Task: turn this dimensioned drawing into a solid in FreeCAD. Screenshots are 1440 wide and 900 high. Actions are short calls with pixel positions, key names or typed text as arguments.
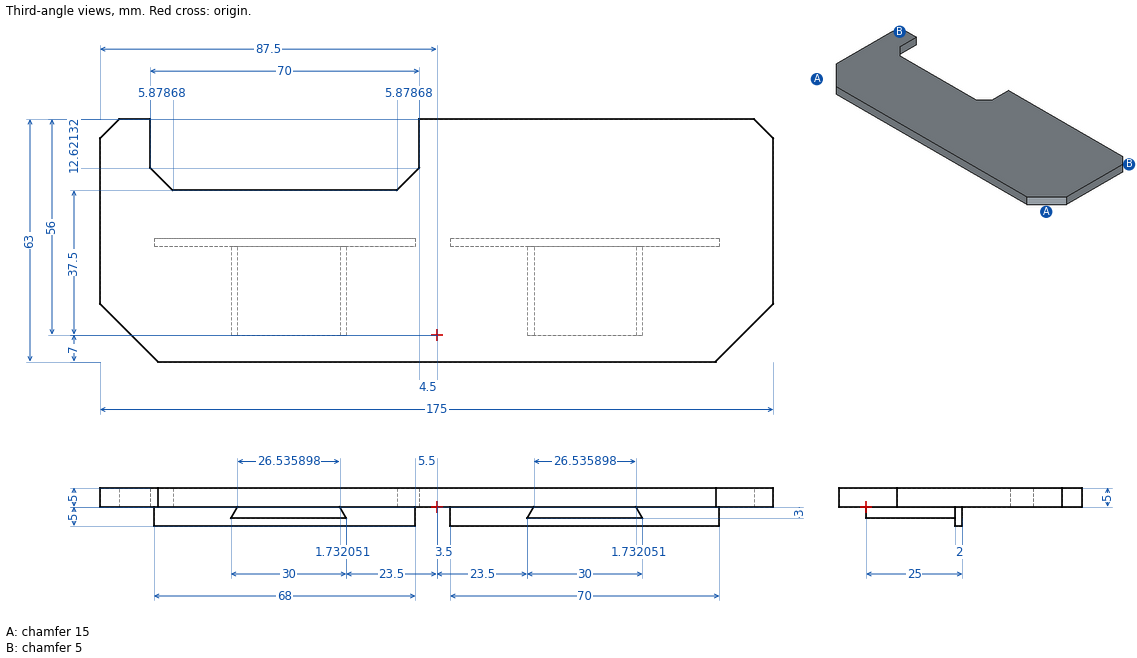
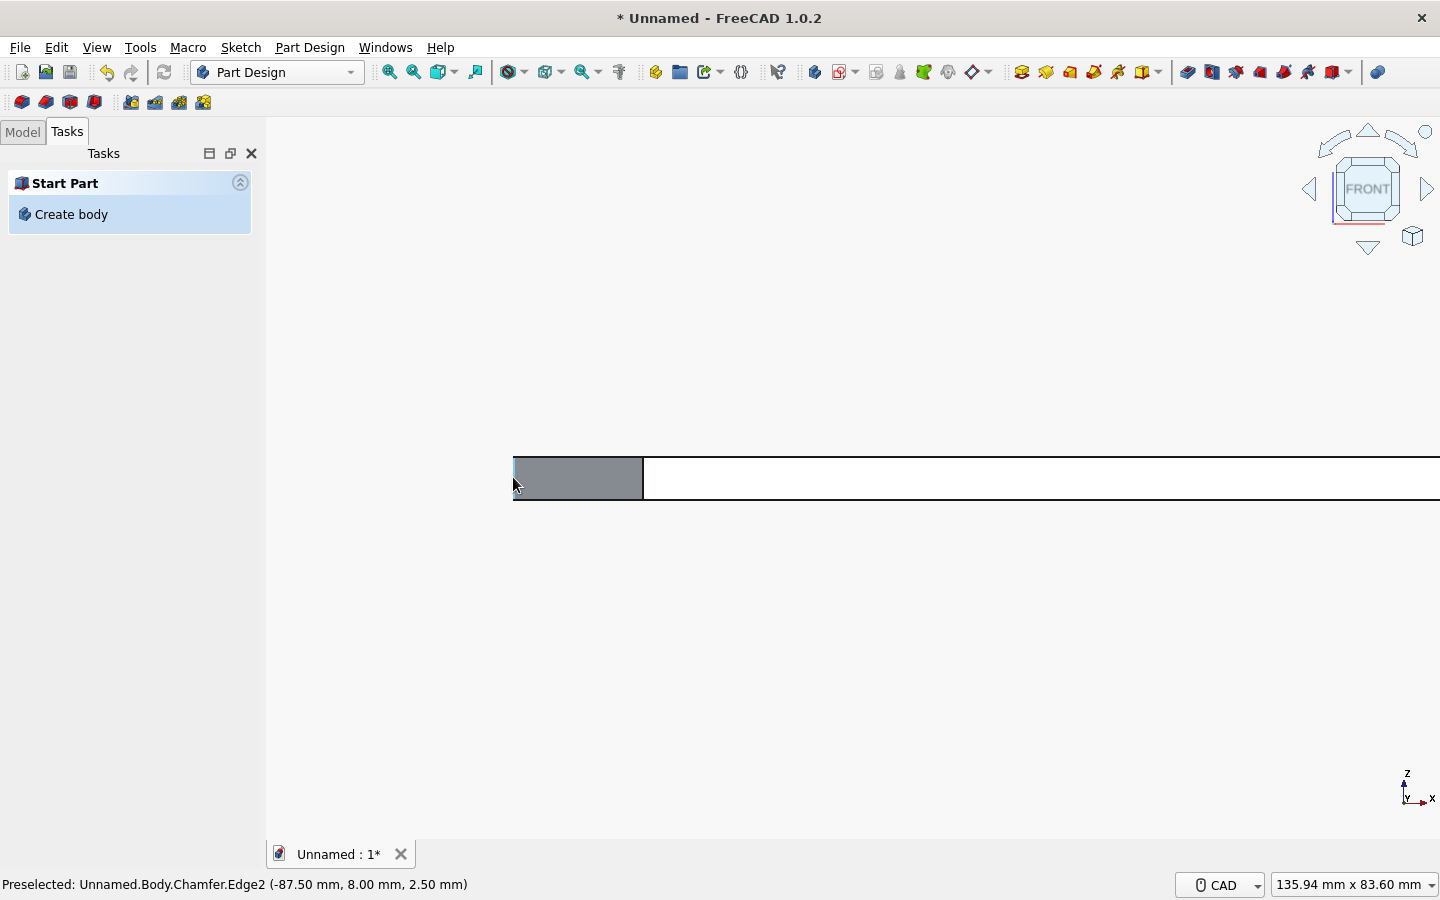
key(v)
key(f)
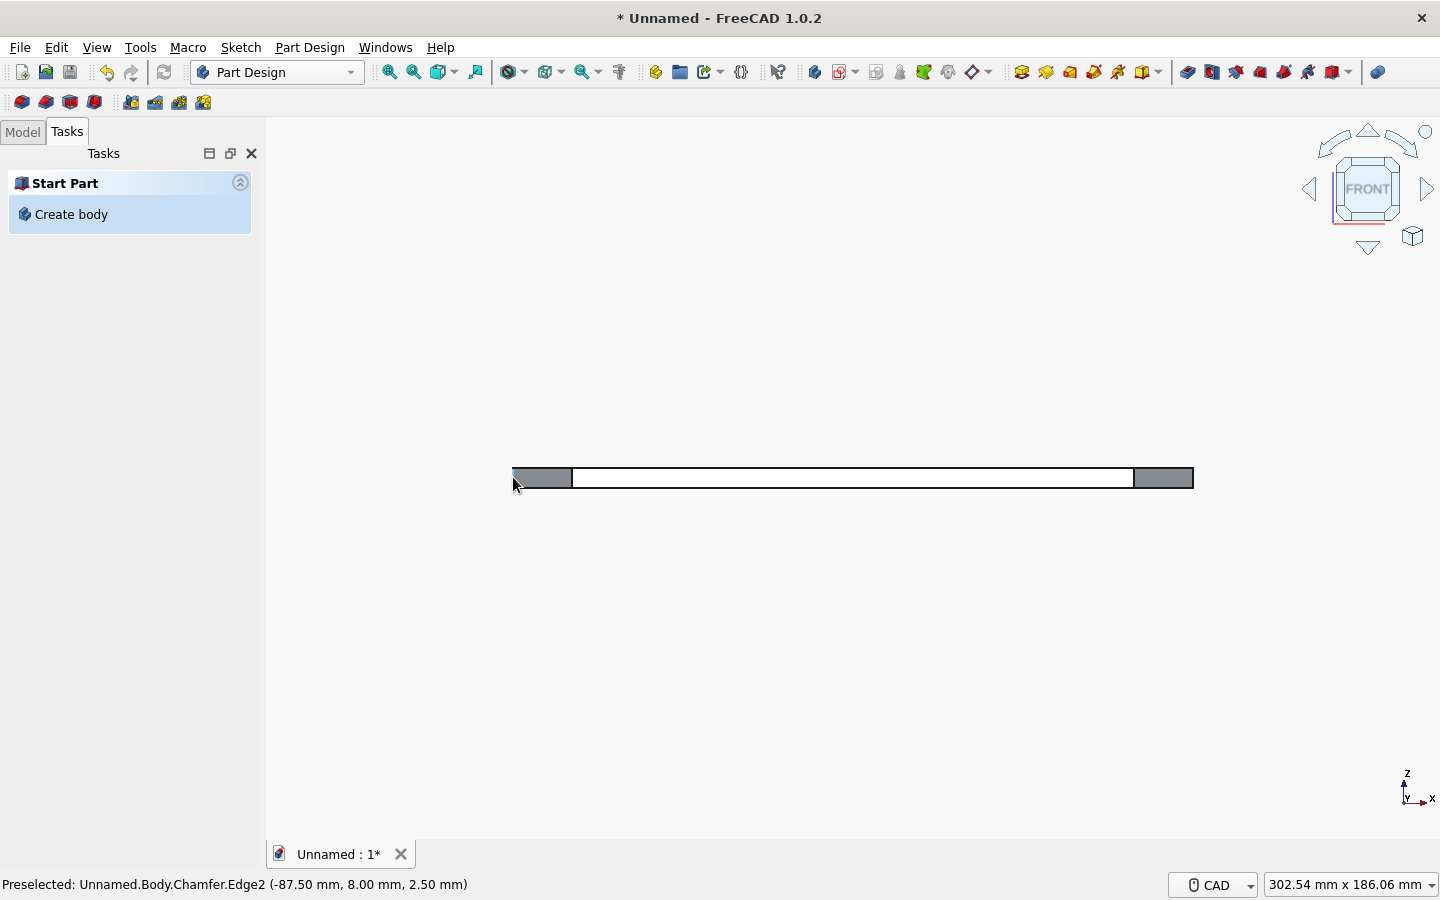
key(0)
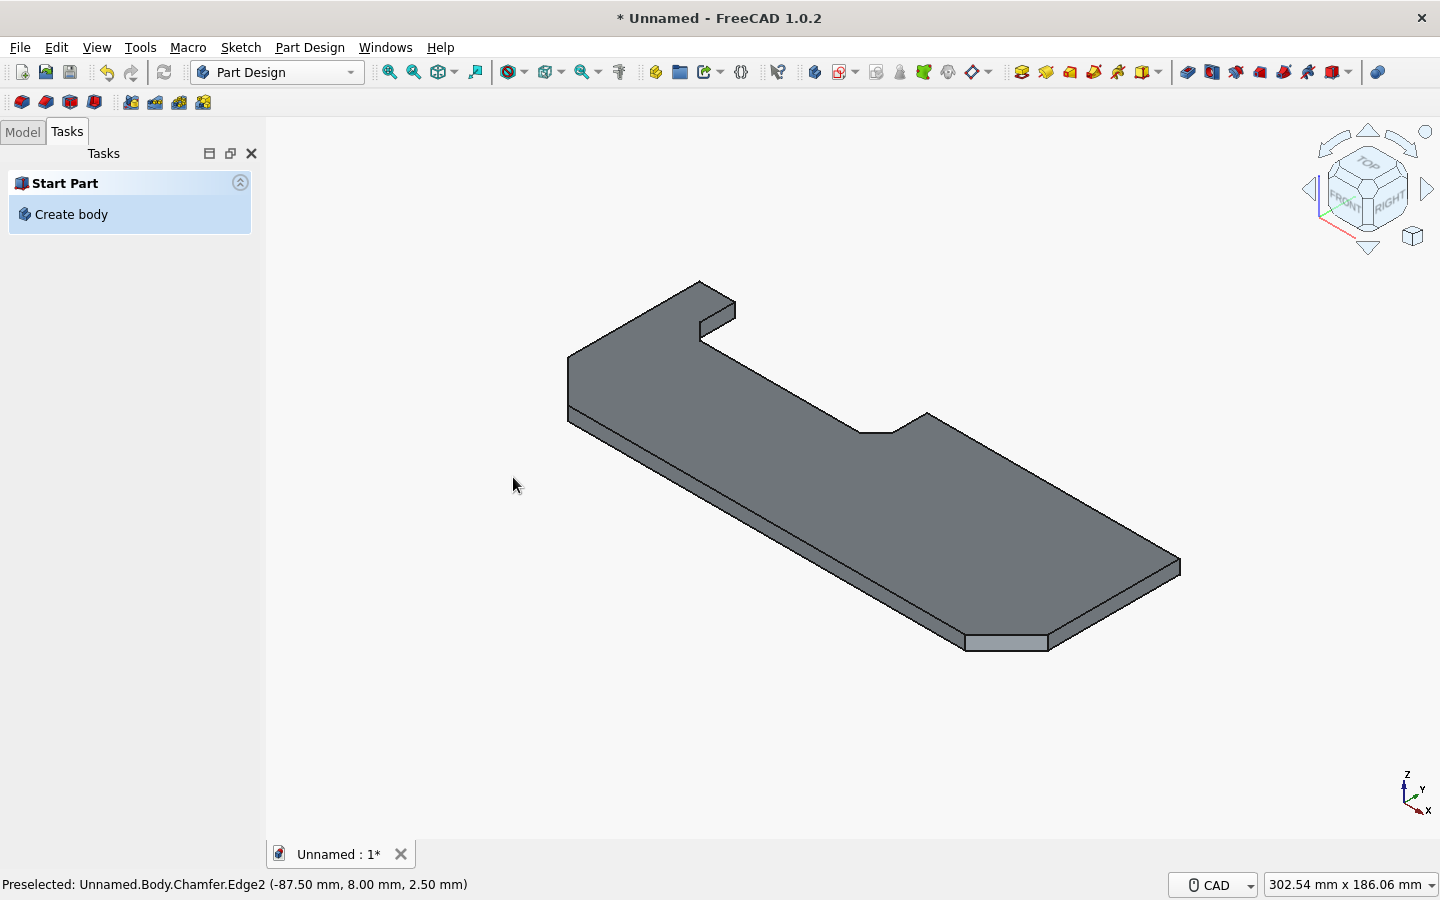
scroll(699, 288, up, 4)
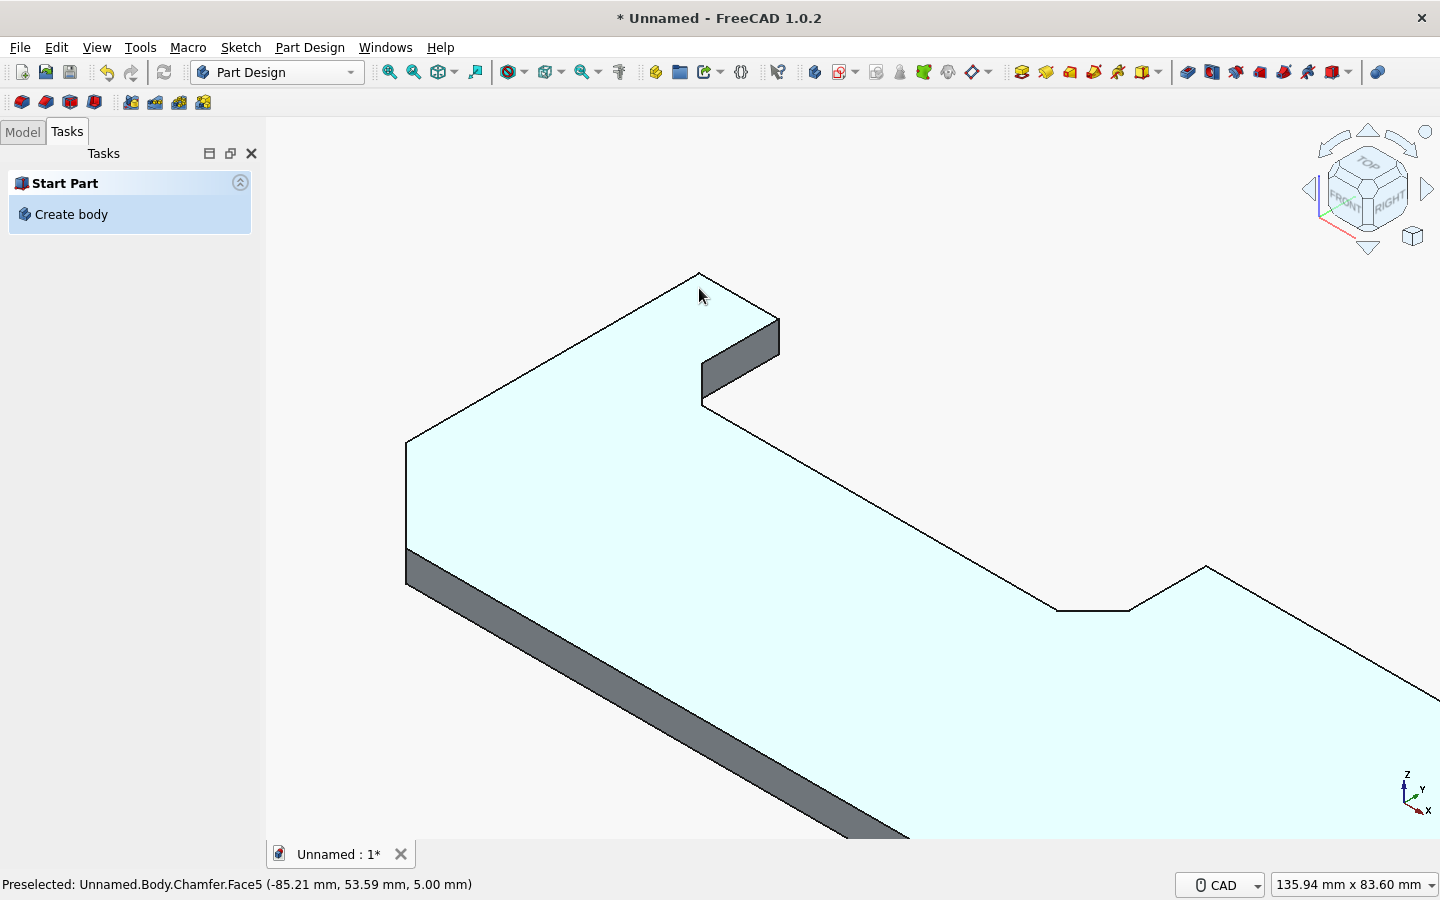
click(390, 72)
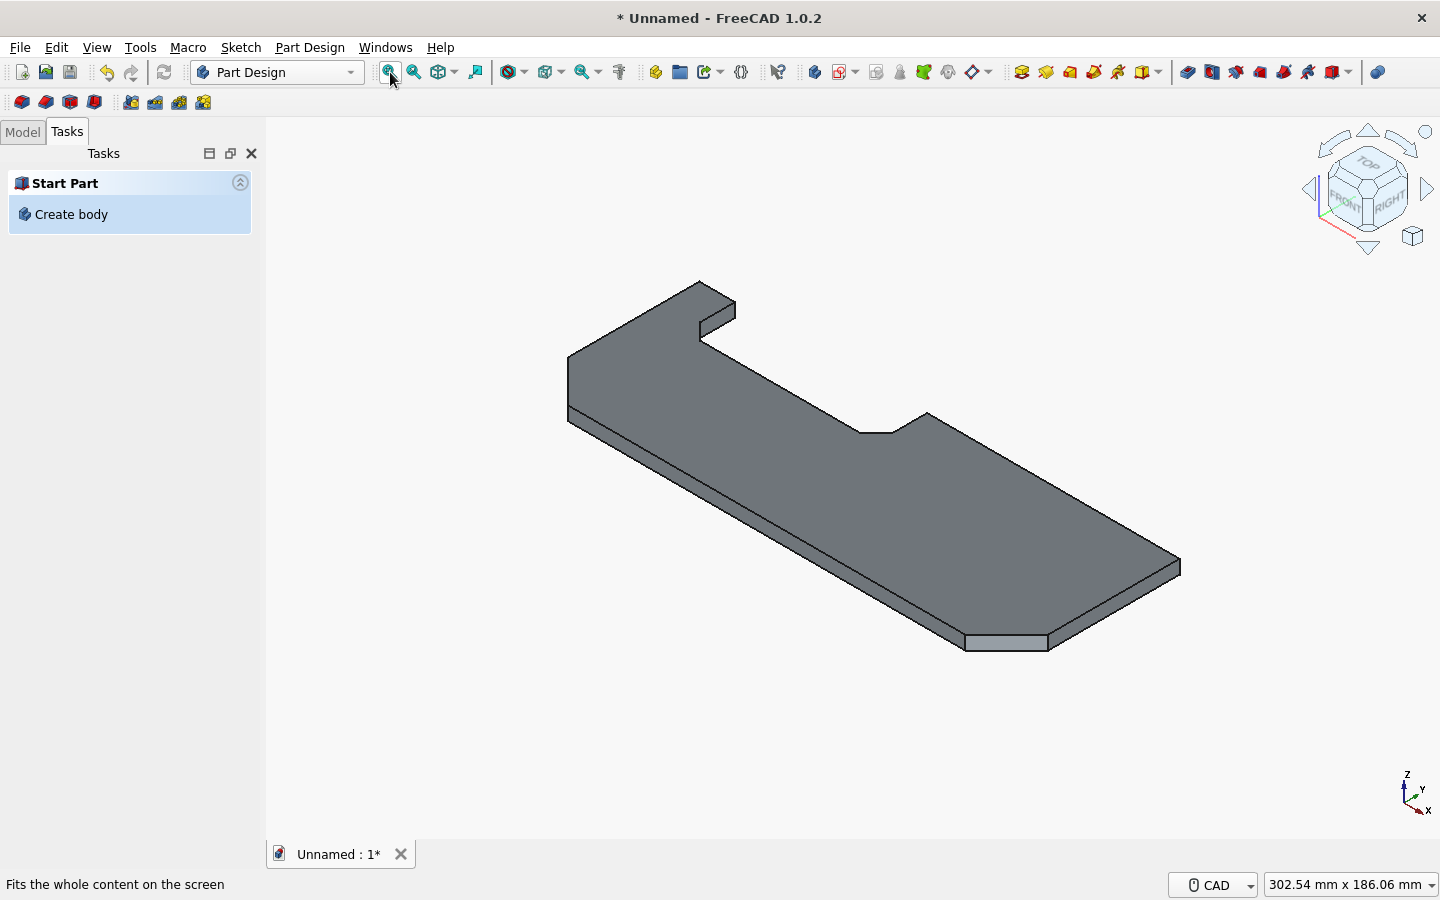
key(2)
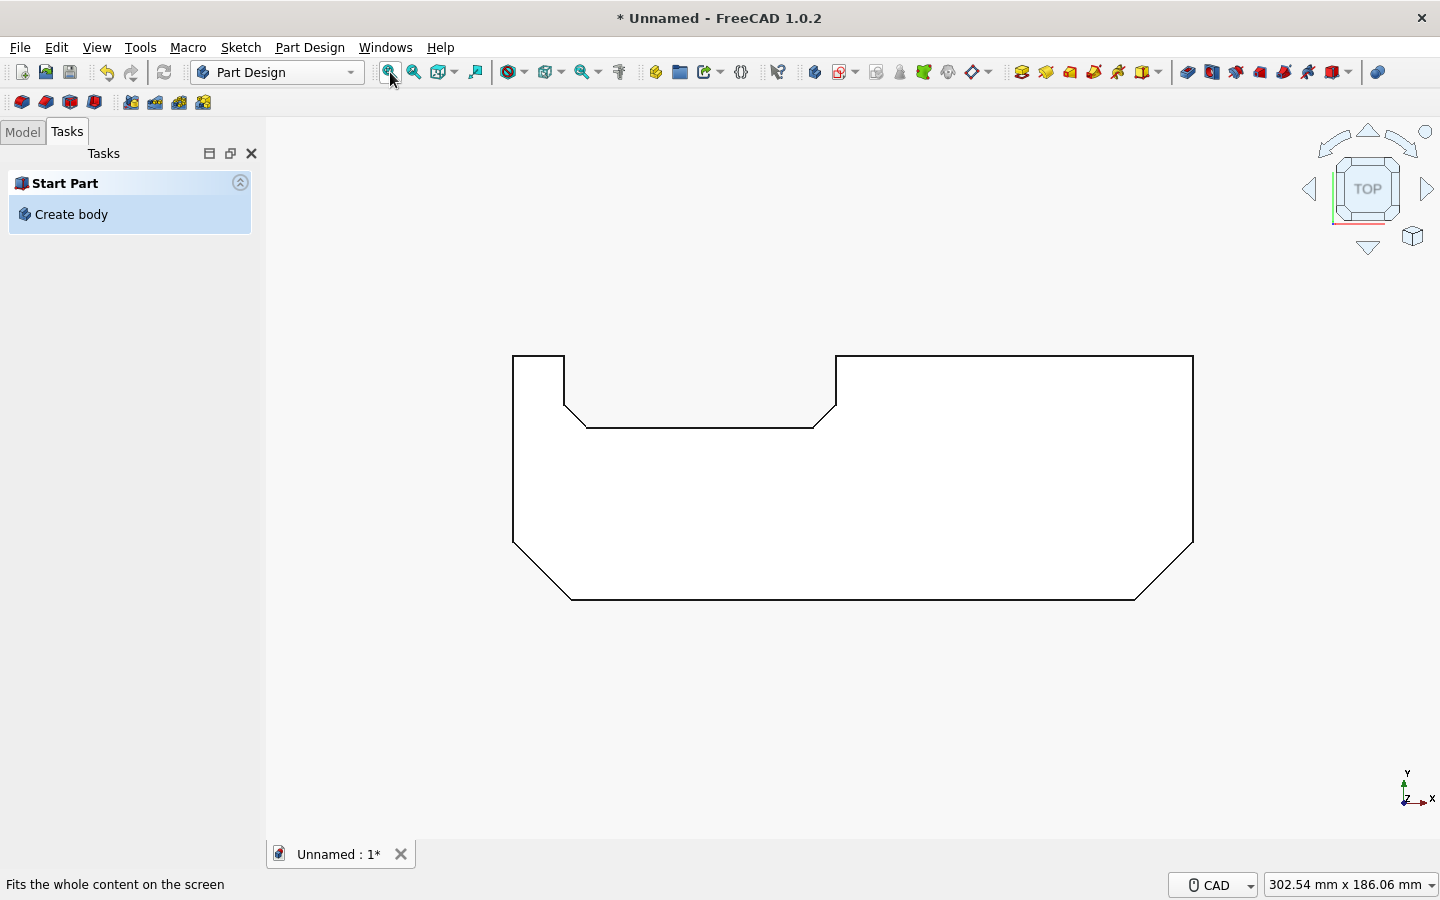
scroll(513, 355, up, 4)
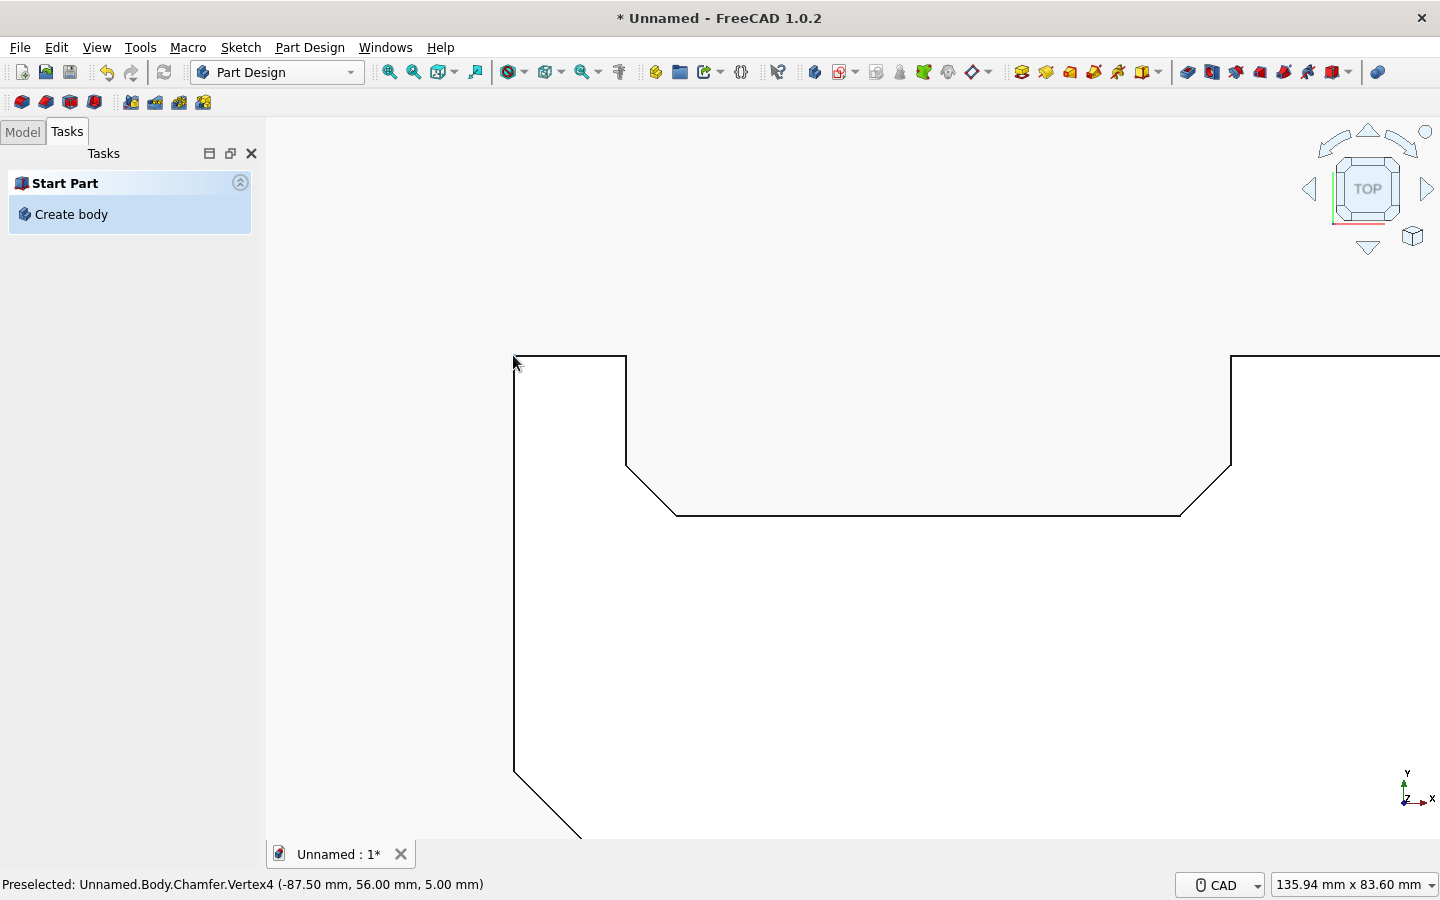
click(390, 72)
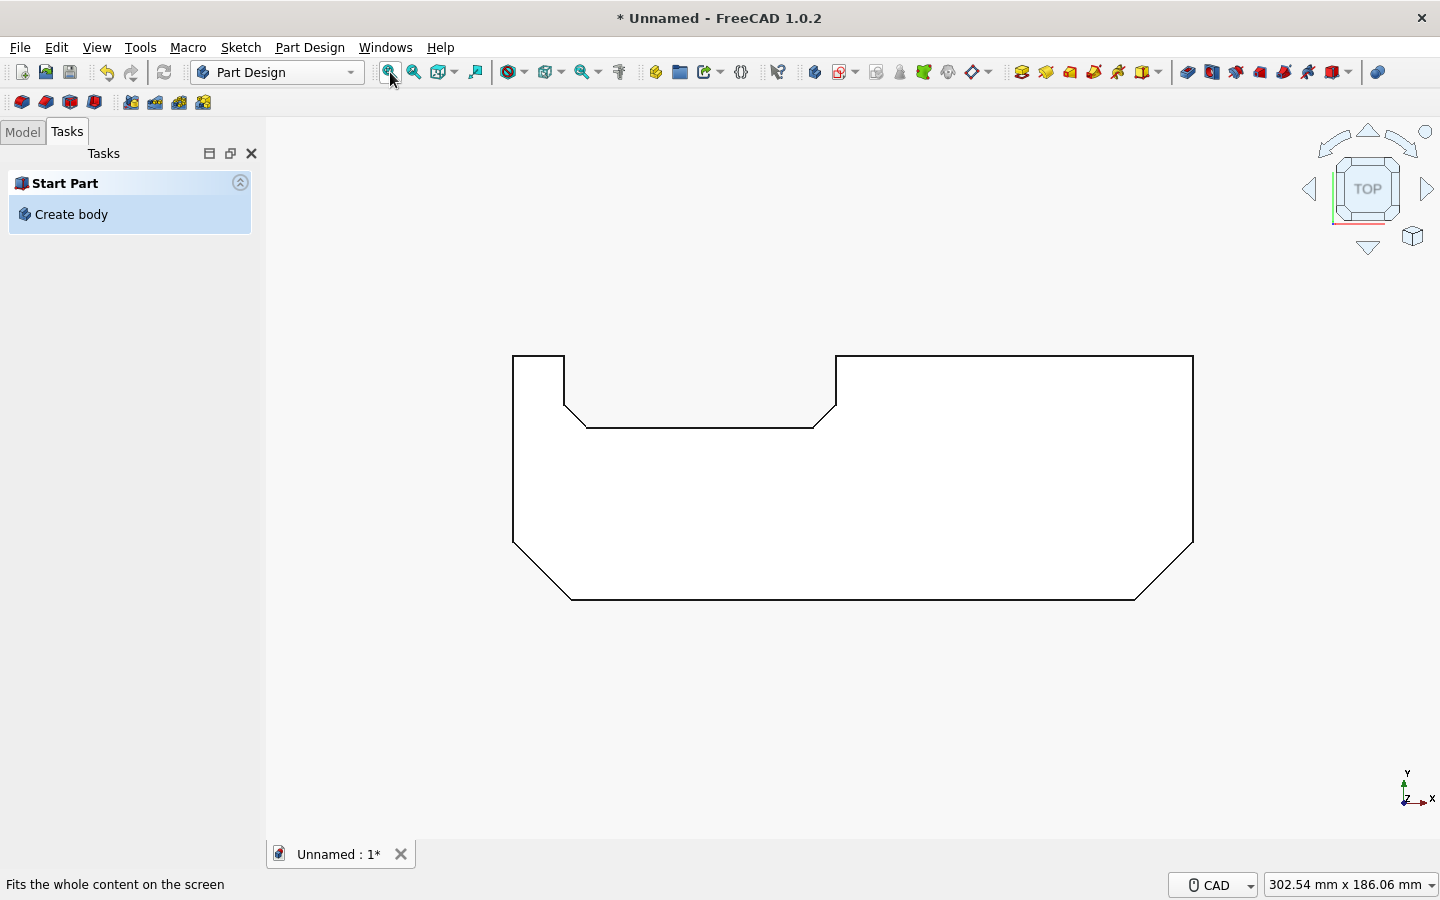
key(1)